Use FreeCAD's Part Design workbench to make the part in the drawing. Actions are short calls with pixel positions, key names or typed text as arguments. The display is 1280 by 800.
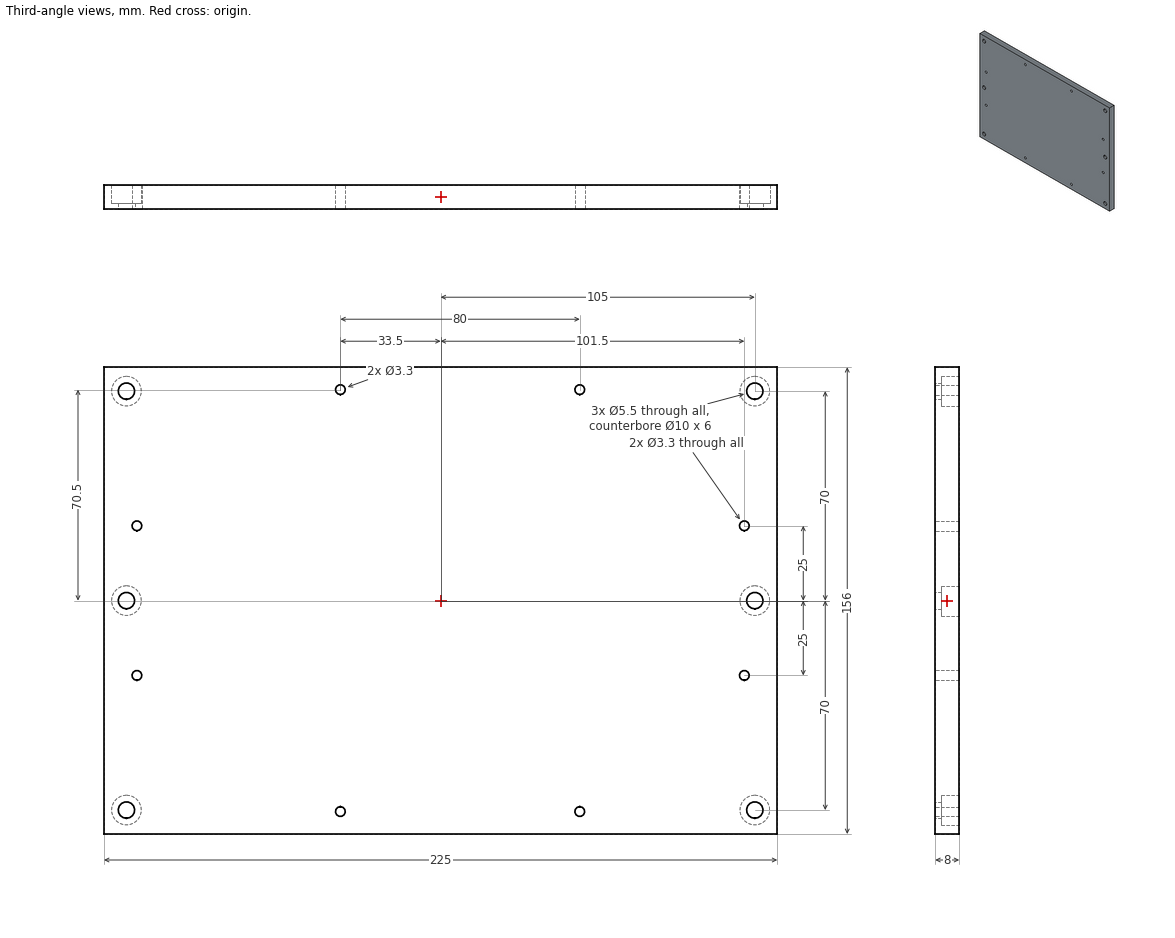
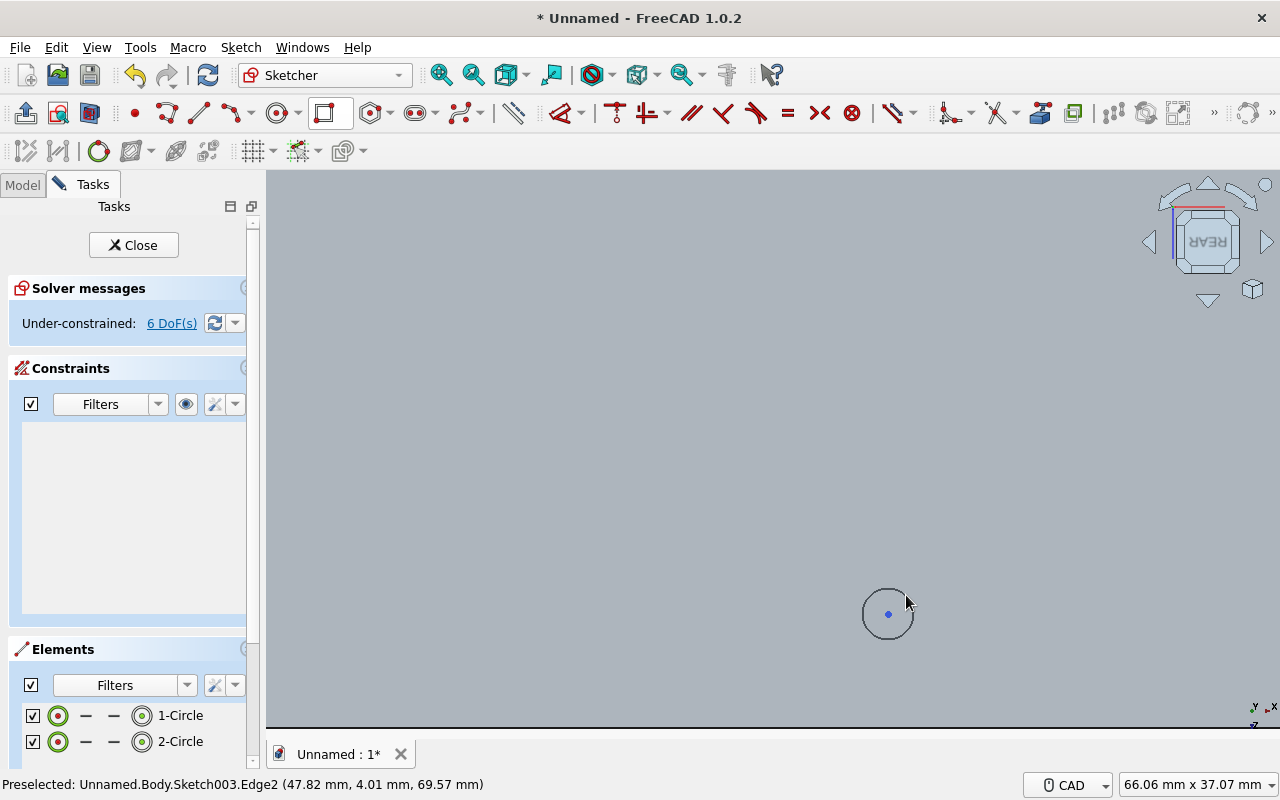
scroll(890, 614, down, 6)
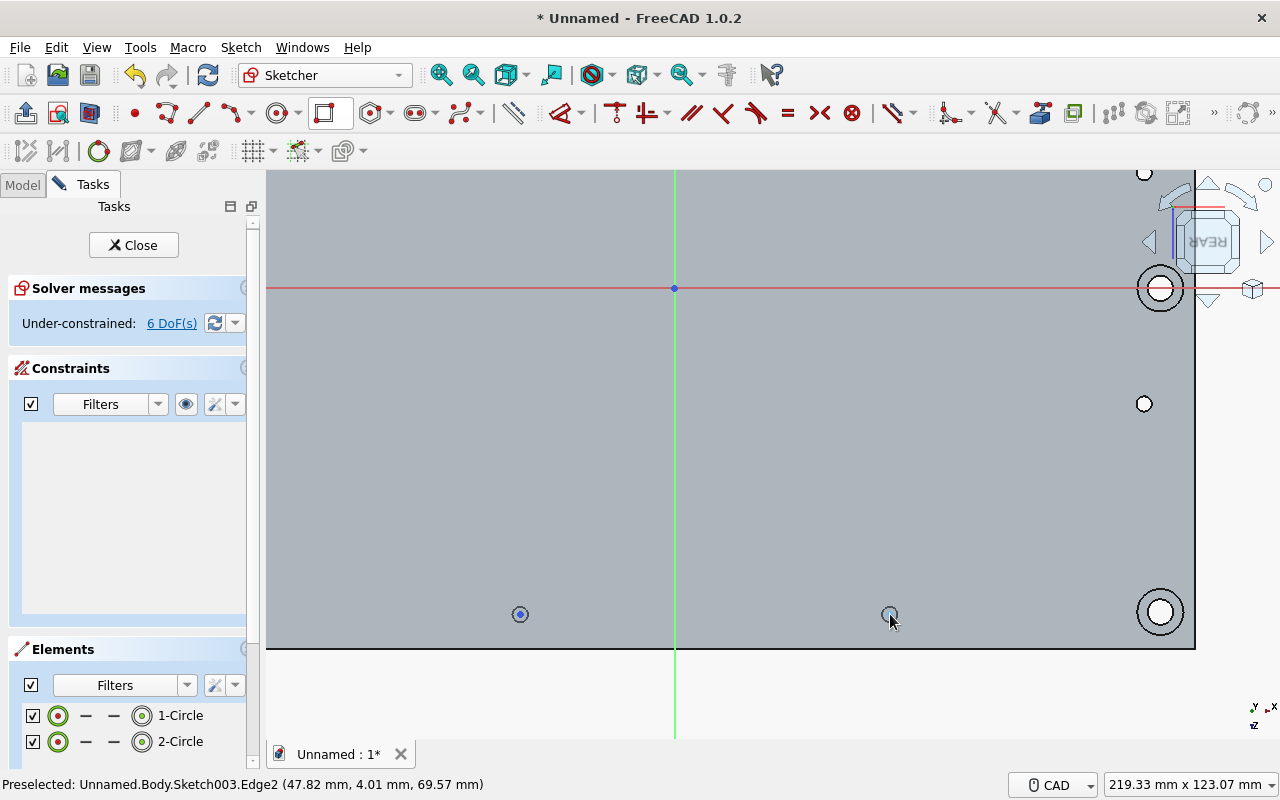
scroll(526, 609, up, 3)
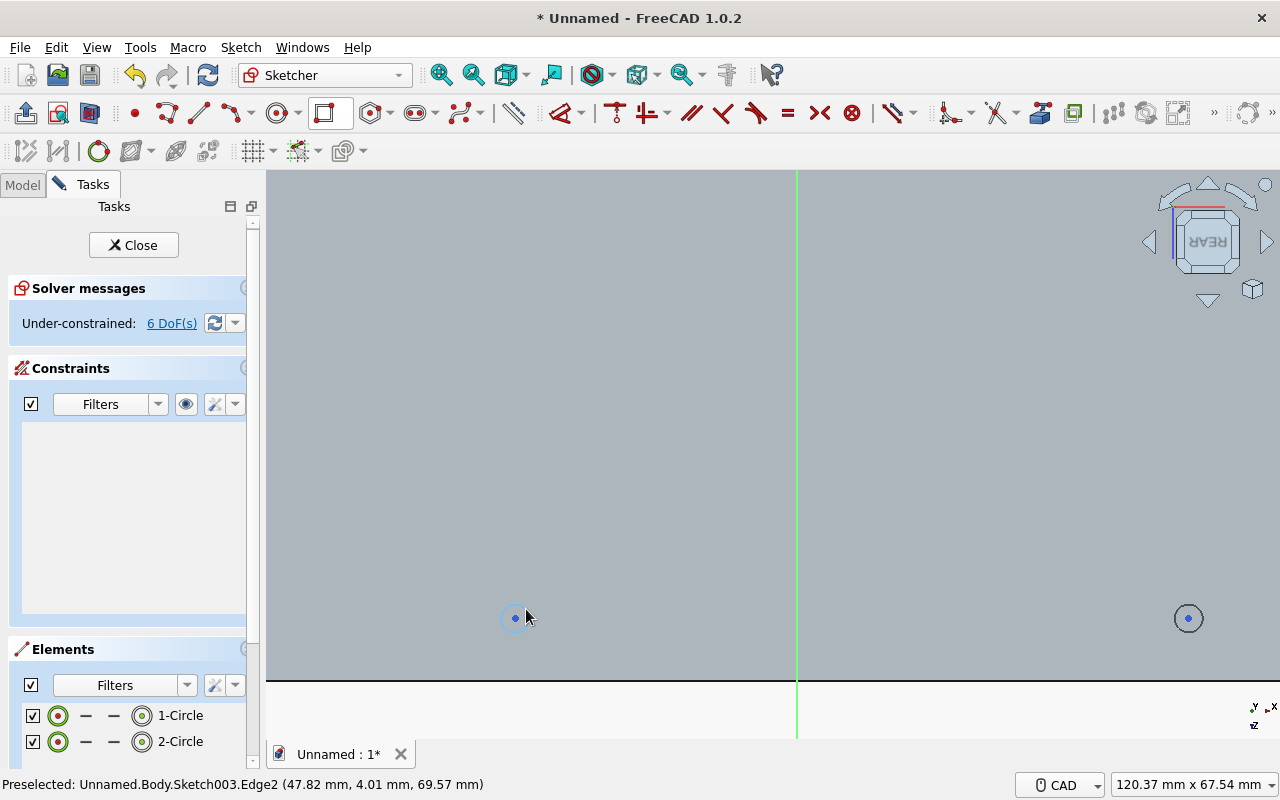
click(525, 609)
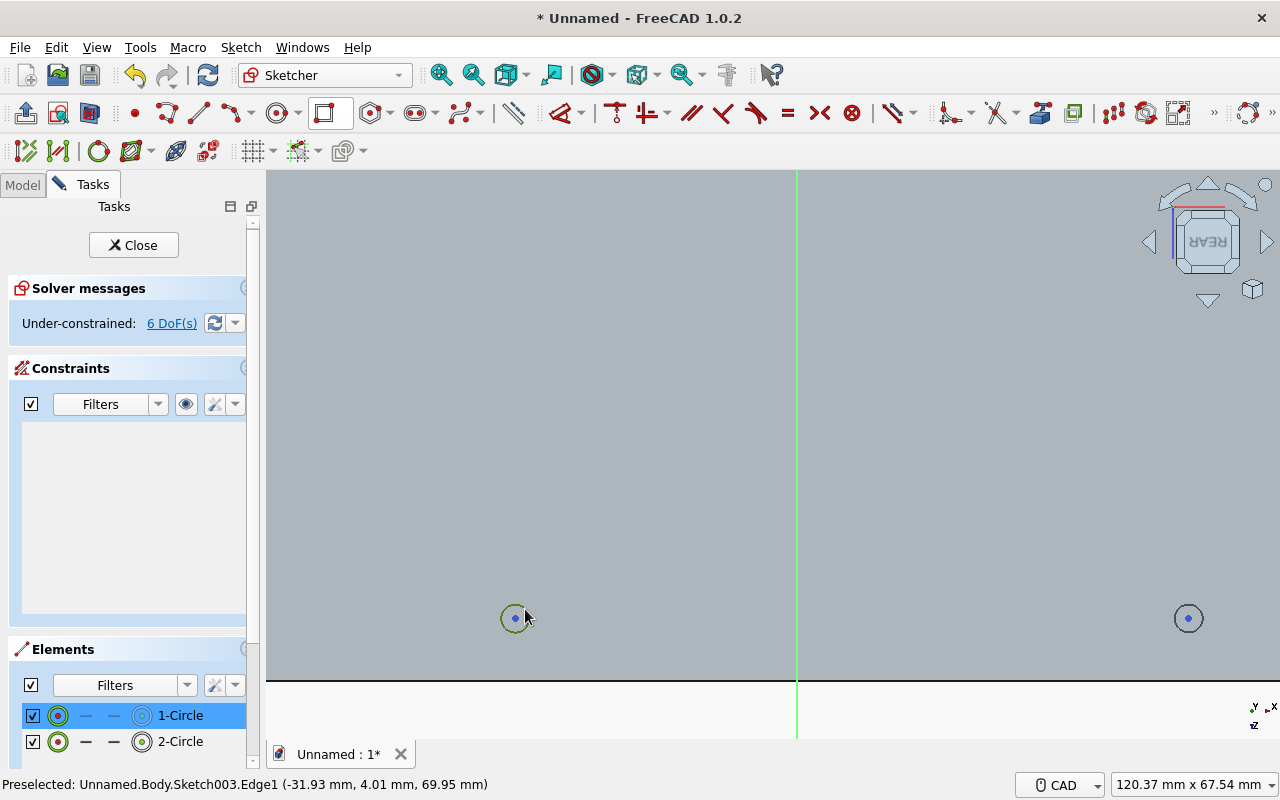
scroll(525, 608, down, 3)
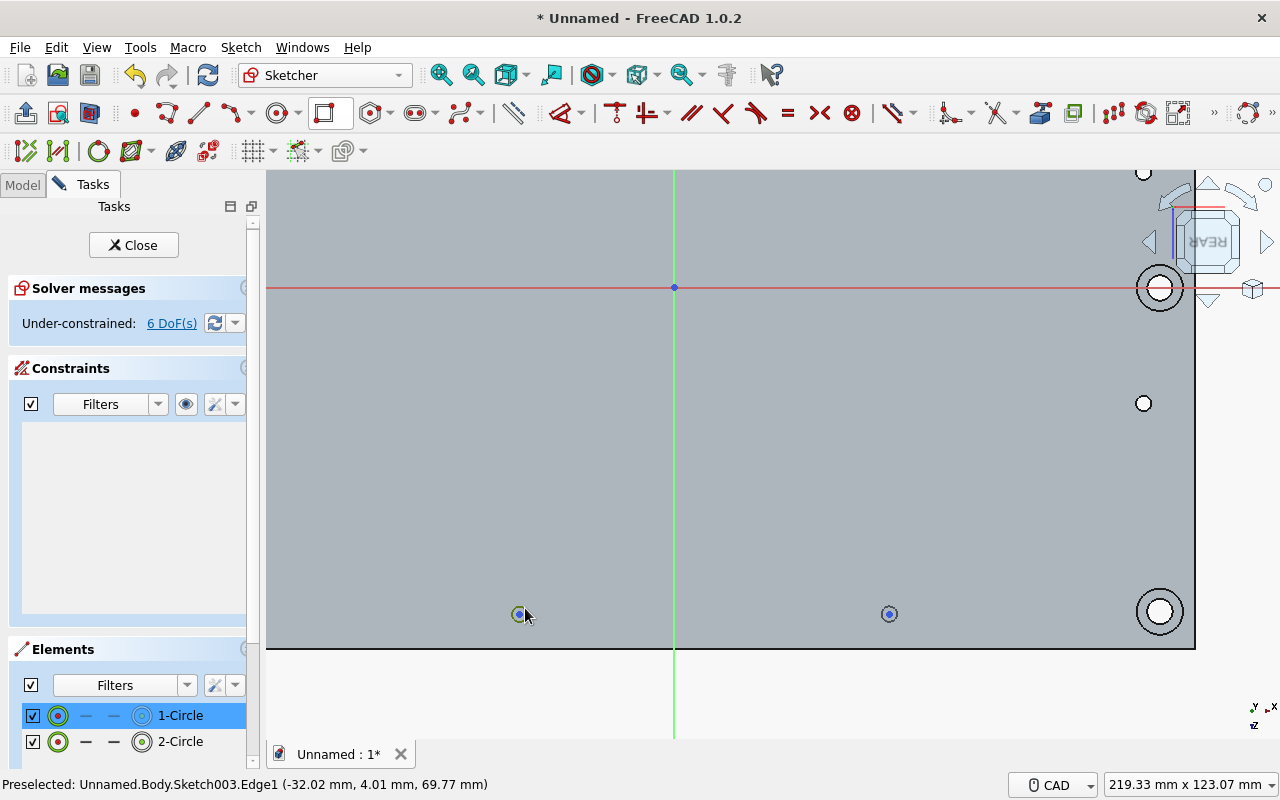
scroll(895, 609, up, 3)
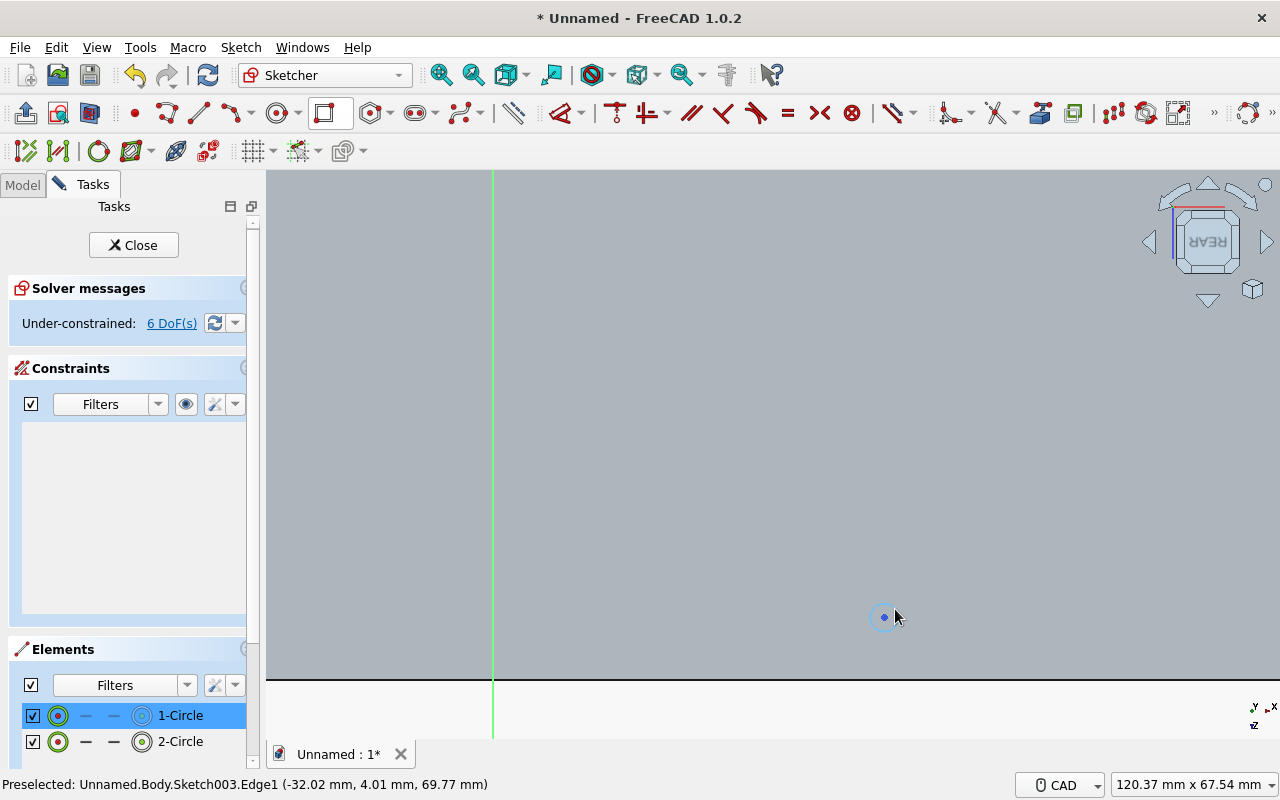
click(894, 608)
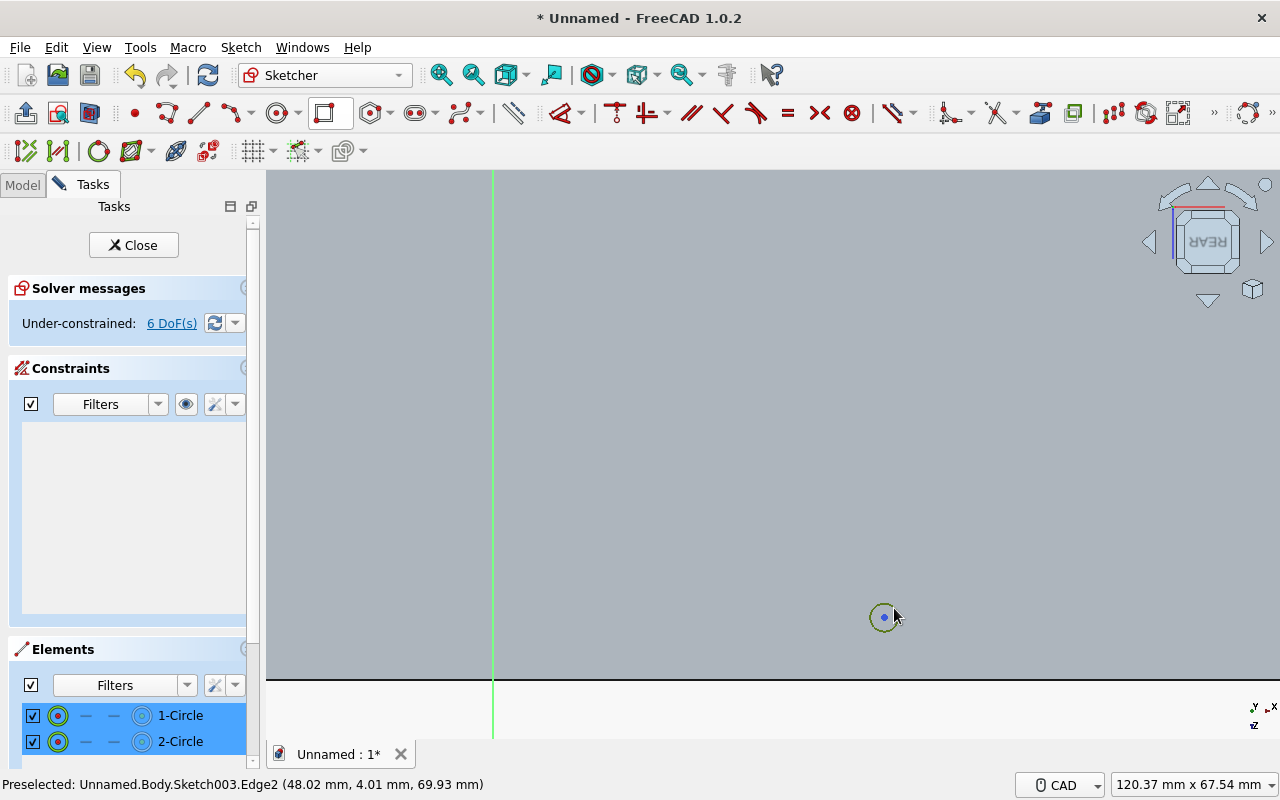
key(e)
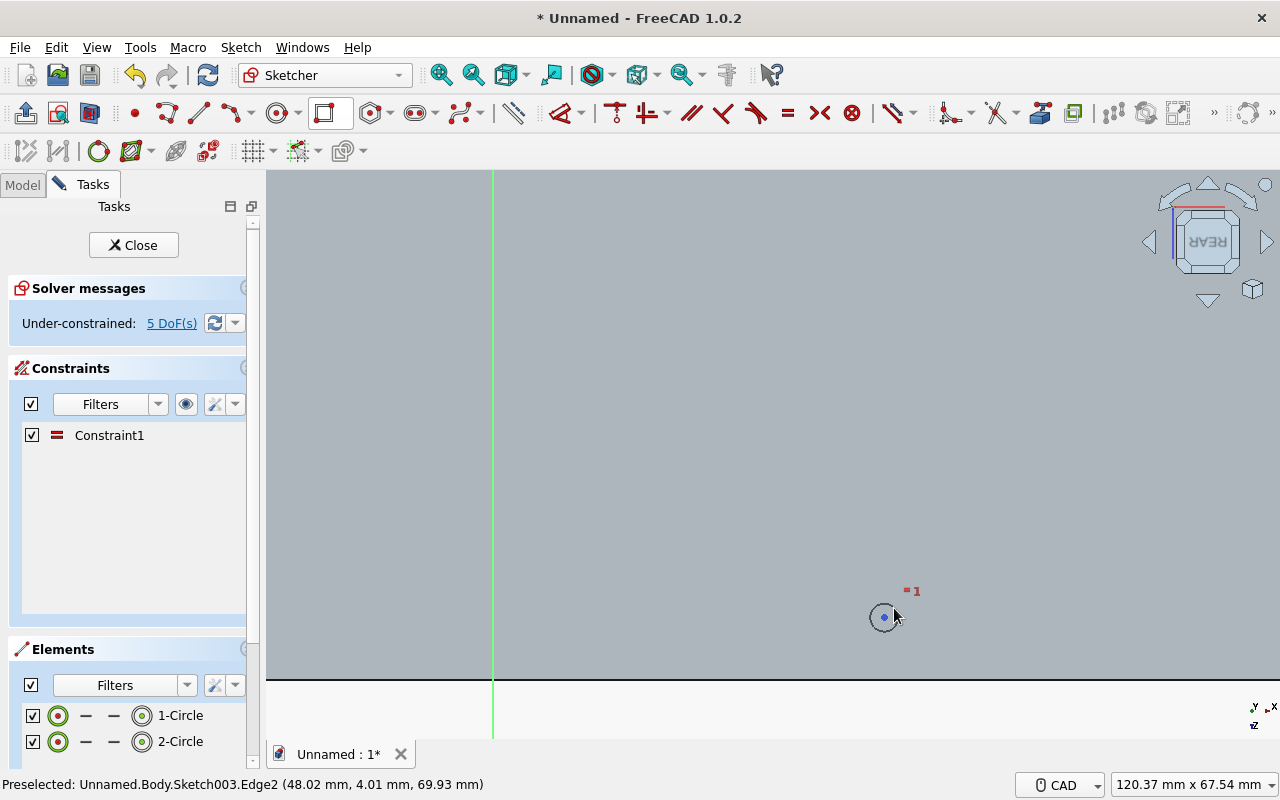
scroll(896, 609, down, 3)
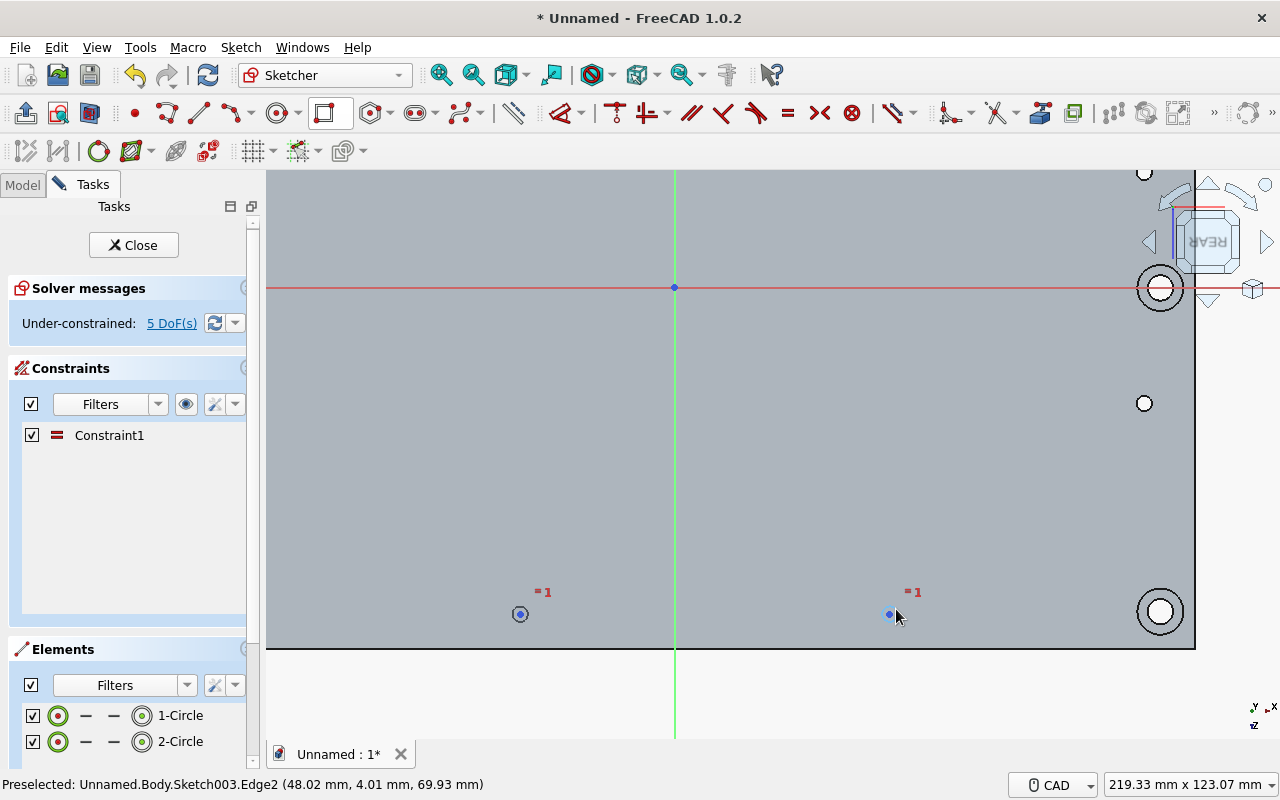
click(520, 614)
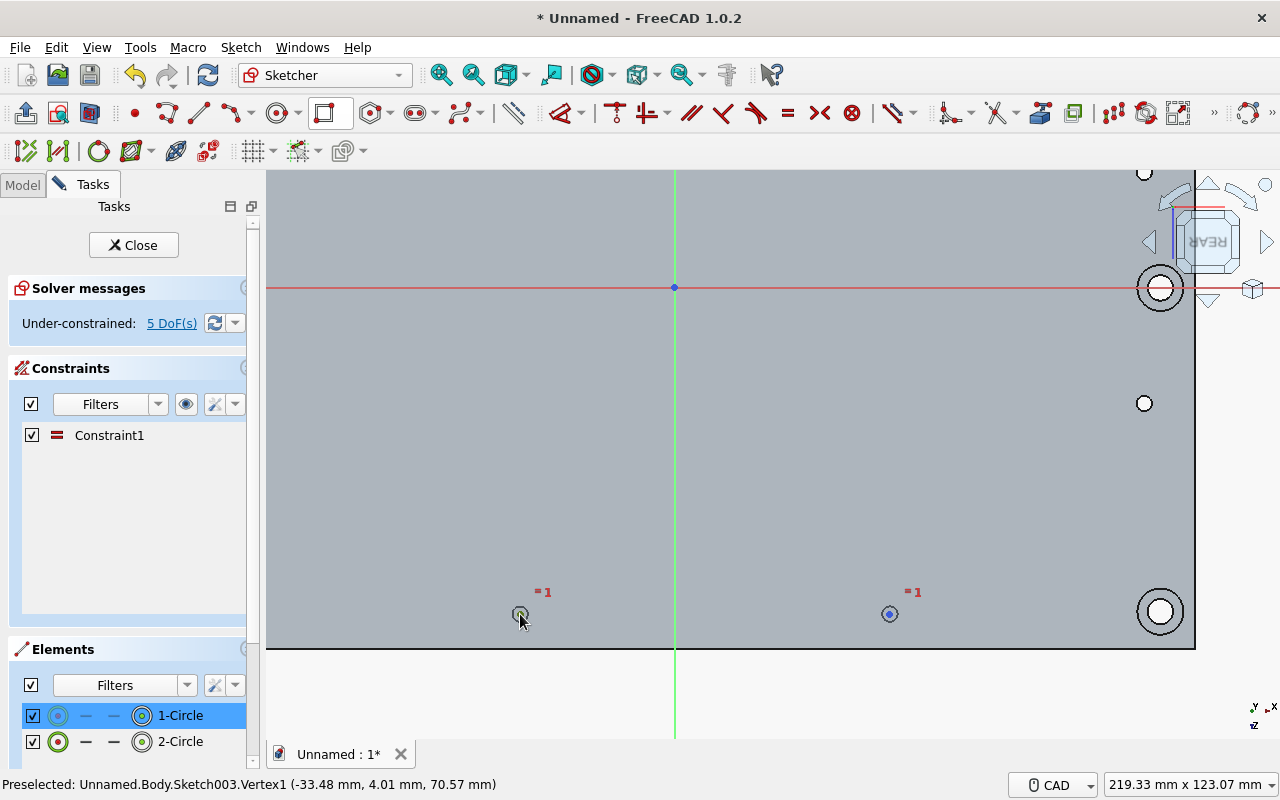
click(890, 614)